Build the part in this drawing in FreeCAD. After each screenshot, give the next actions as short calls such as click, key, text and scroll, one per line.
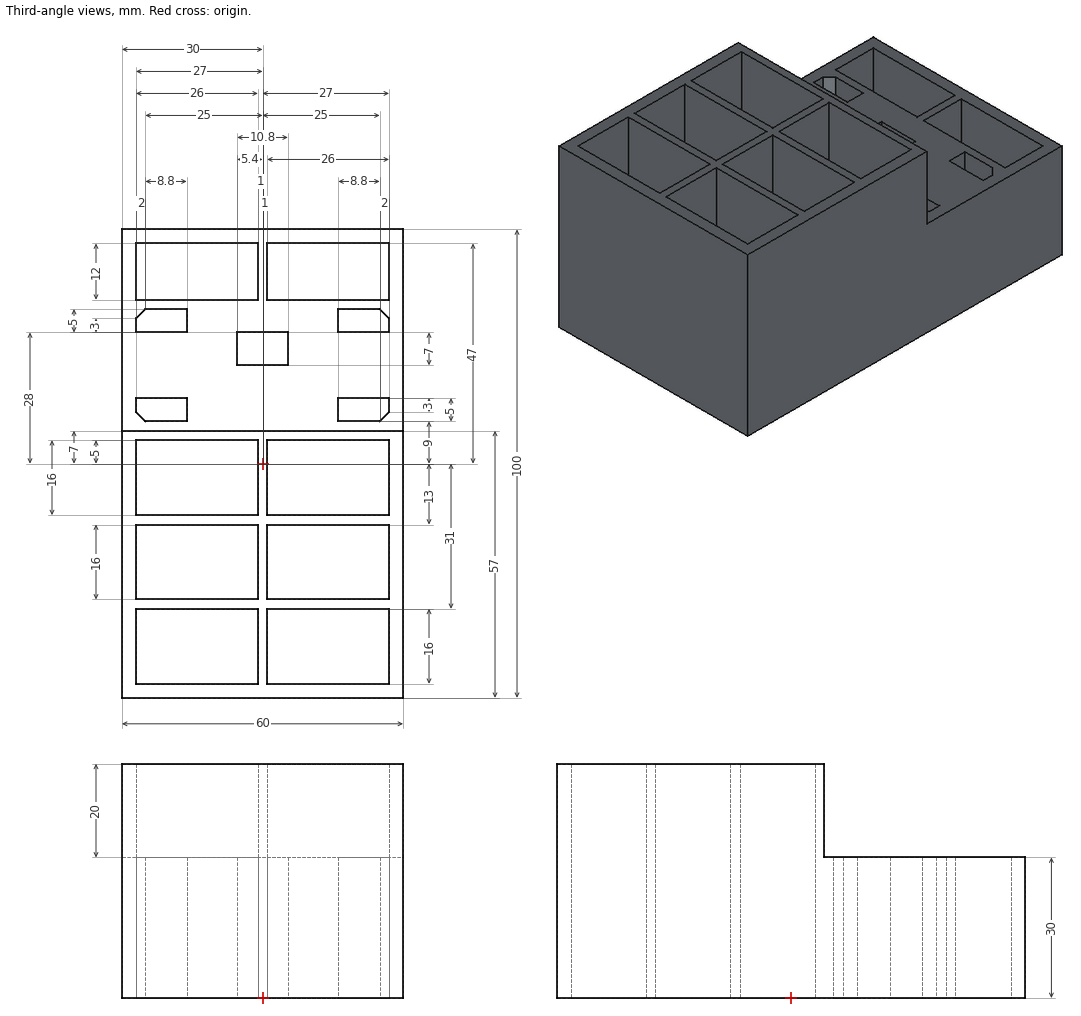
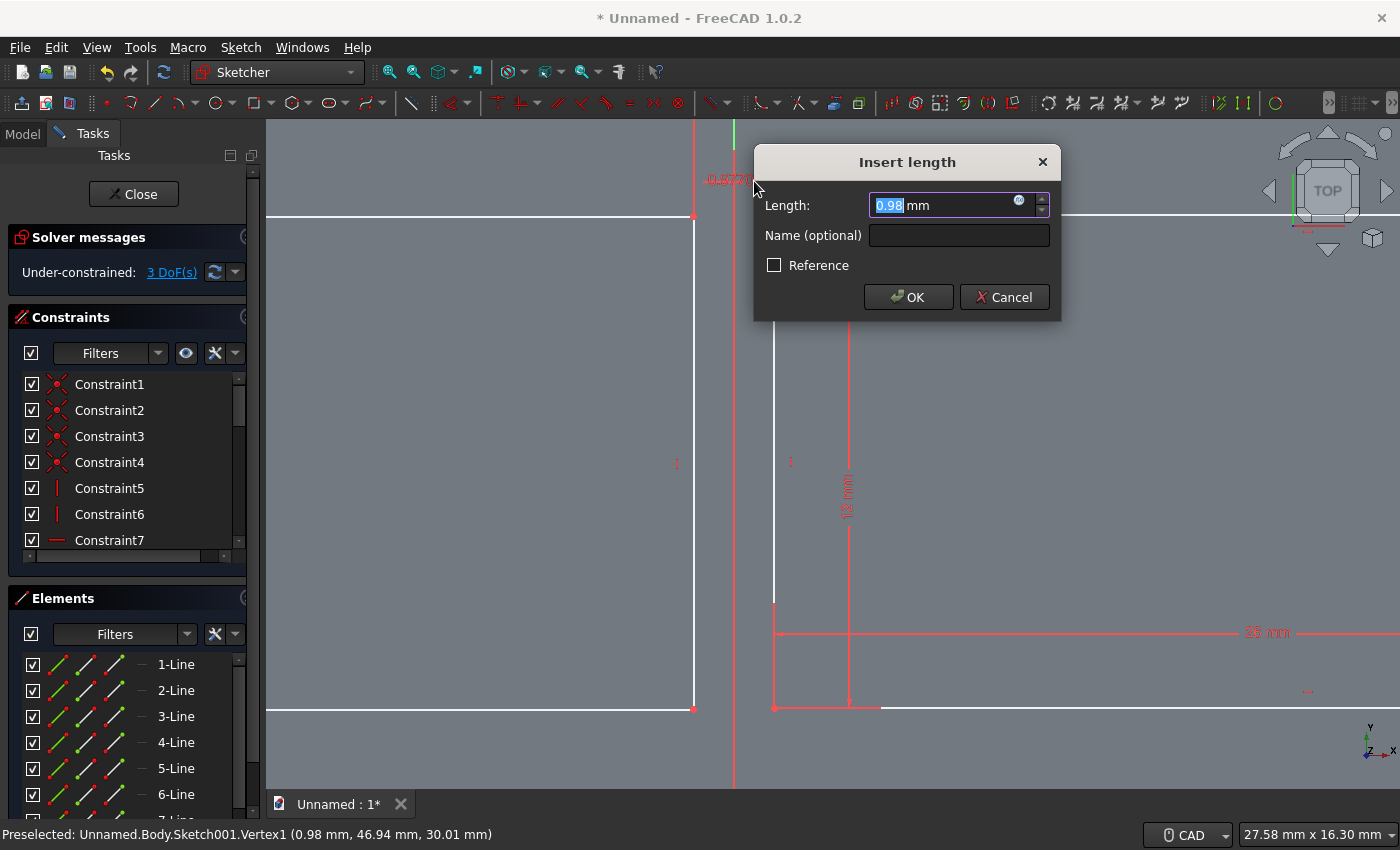
text(1)
key(Return)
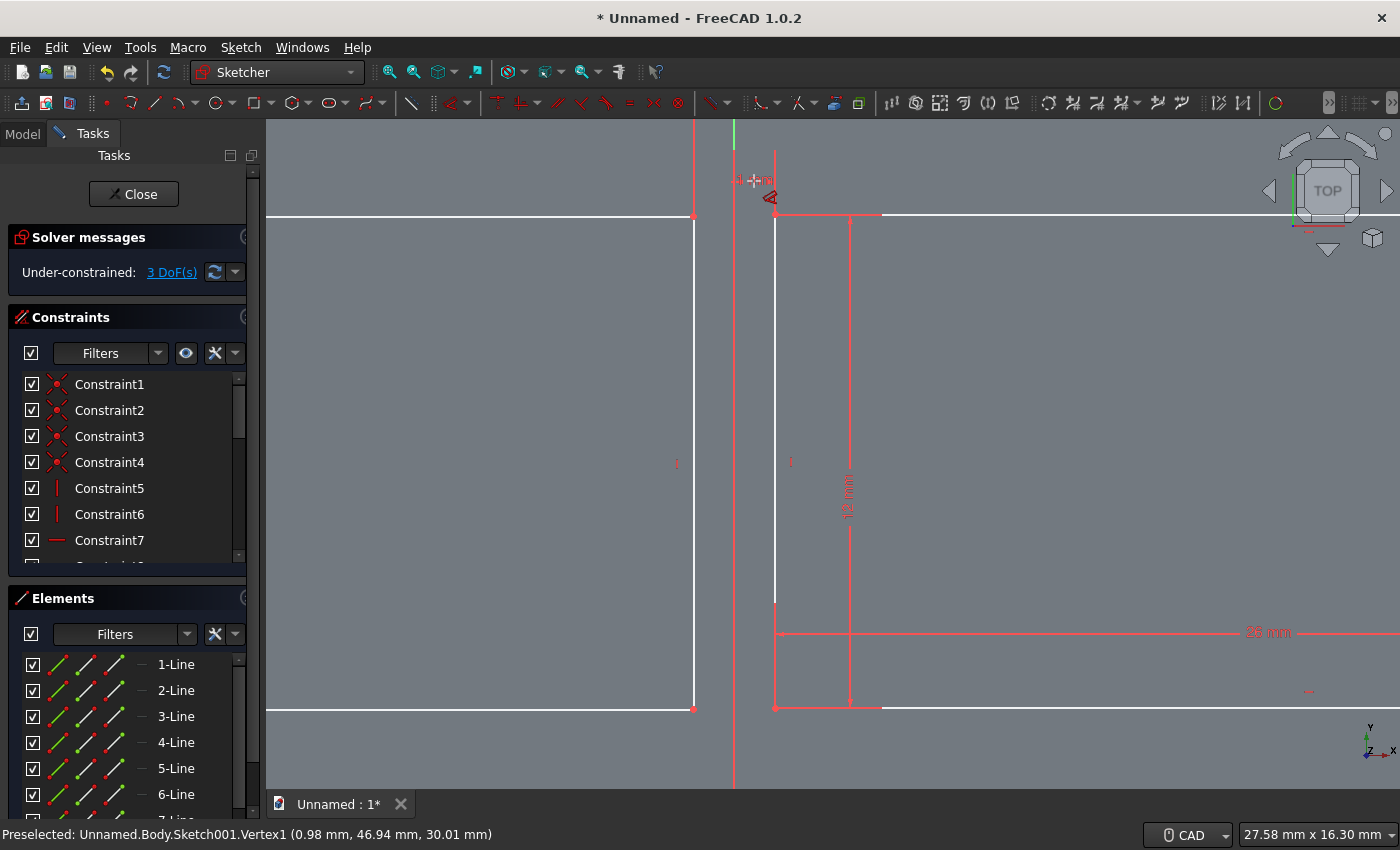
click(694, 710)
click(714, 676)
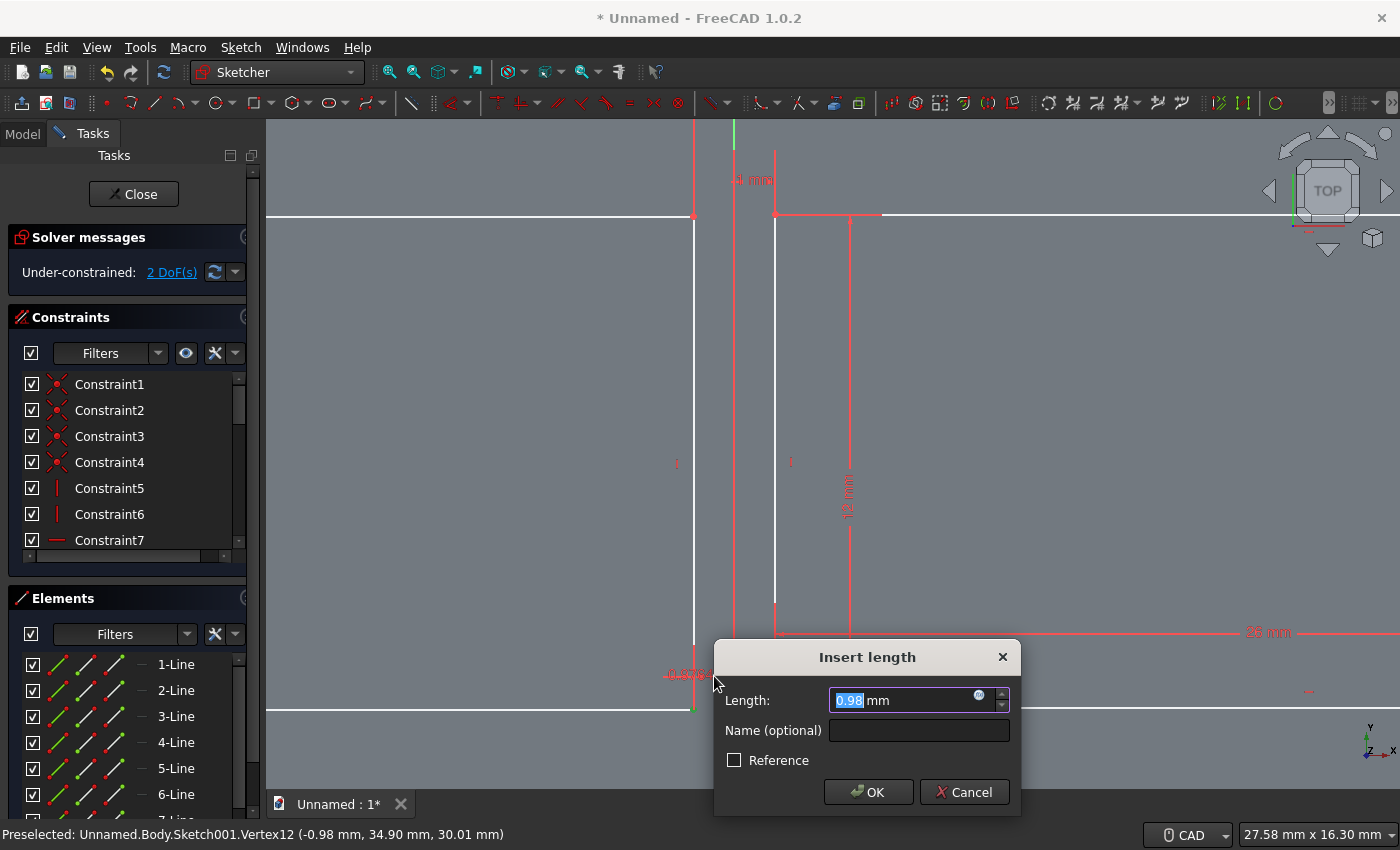
text(1)
key(Return)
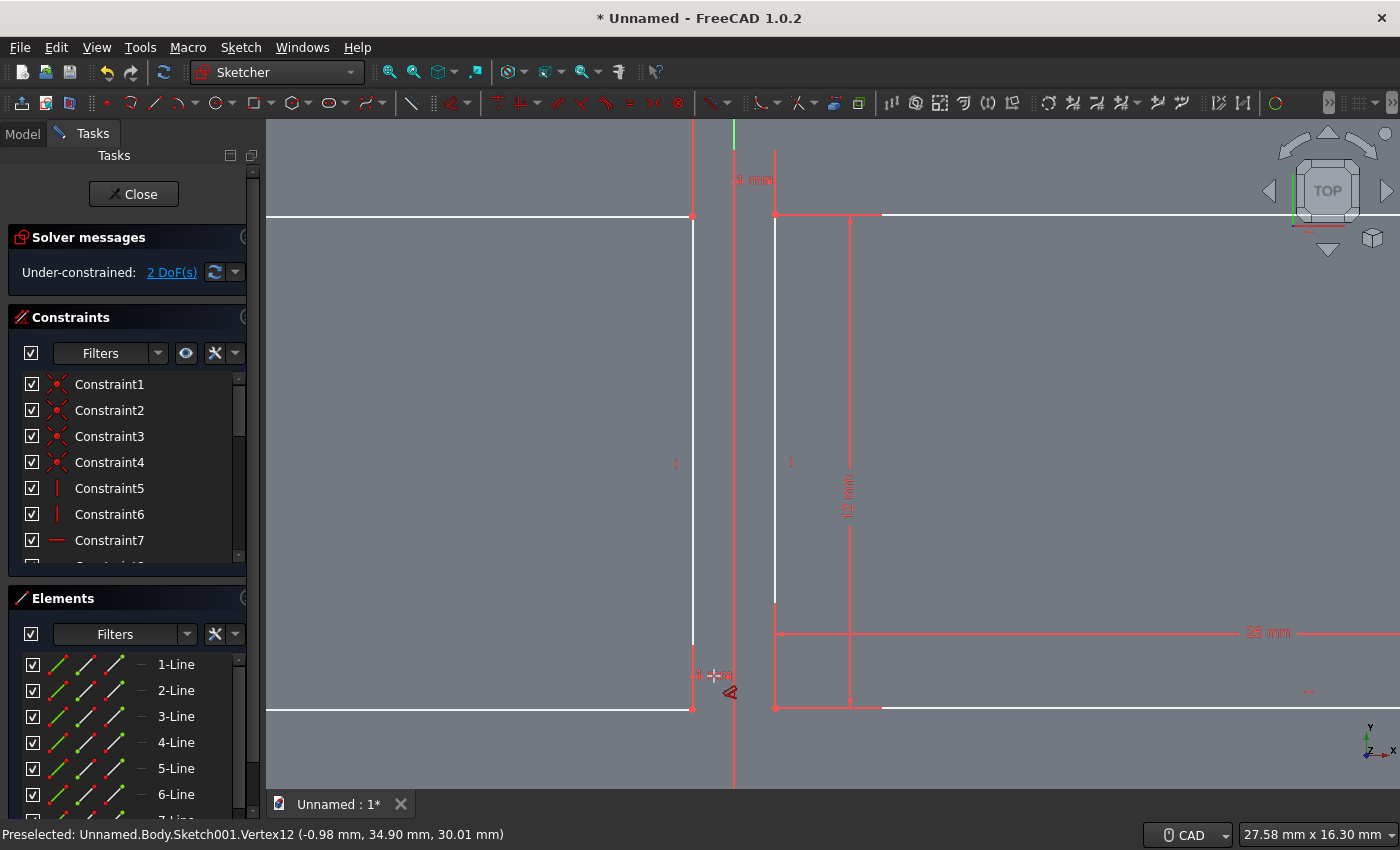
scroll(774, 217, down, 7)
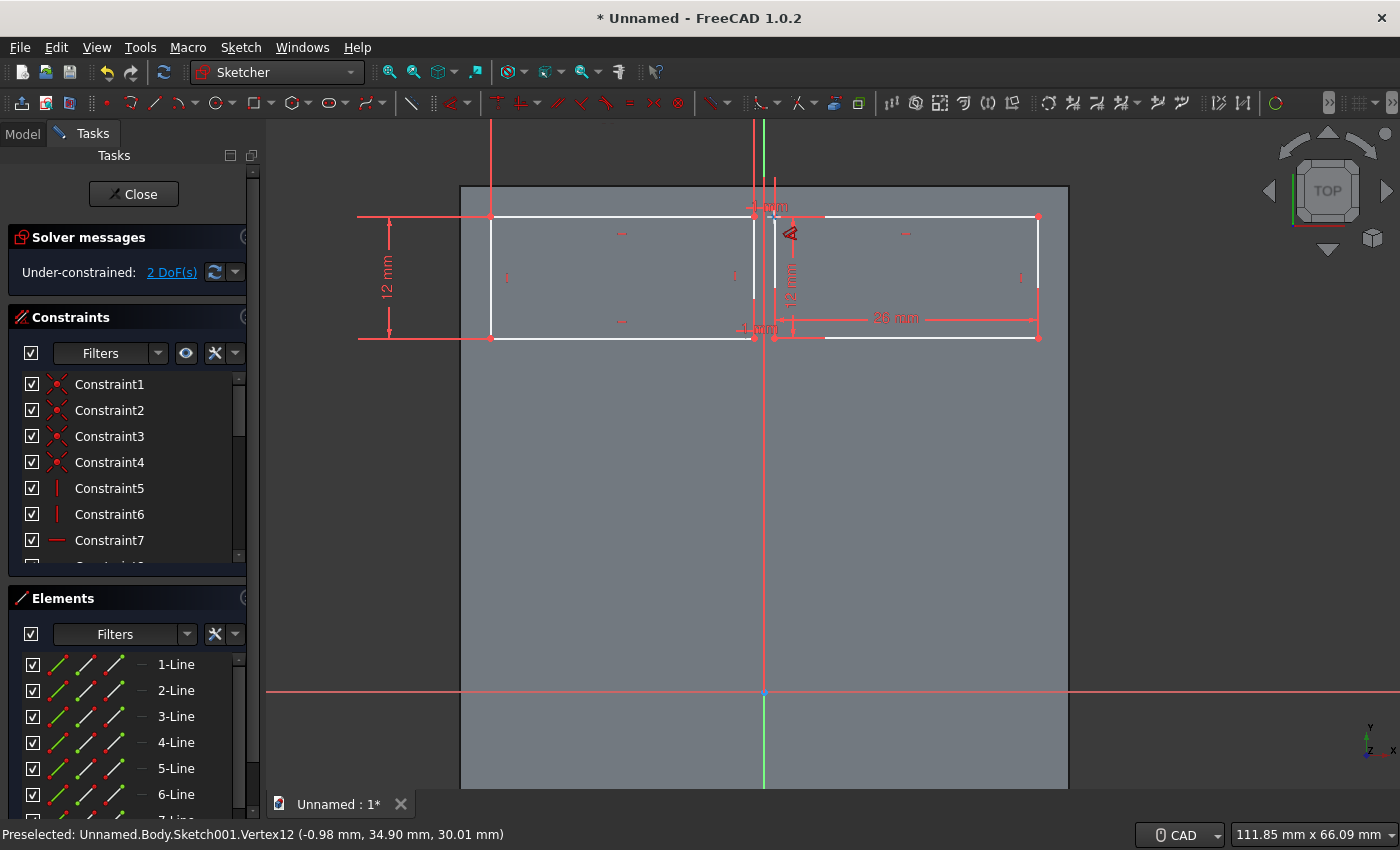
click(775, 217)
click(809, 455)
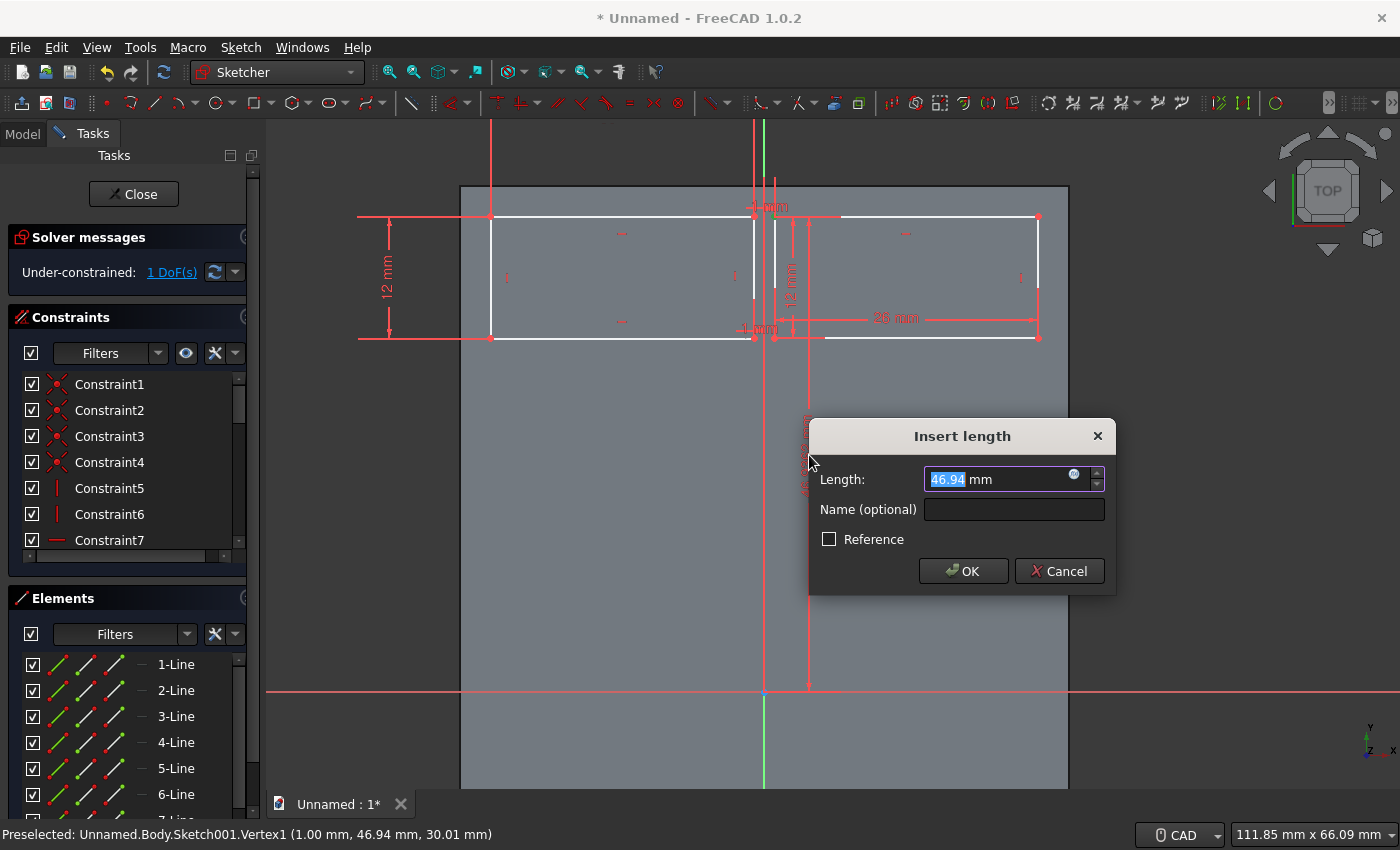
text(47)
key(Return)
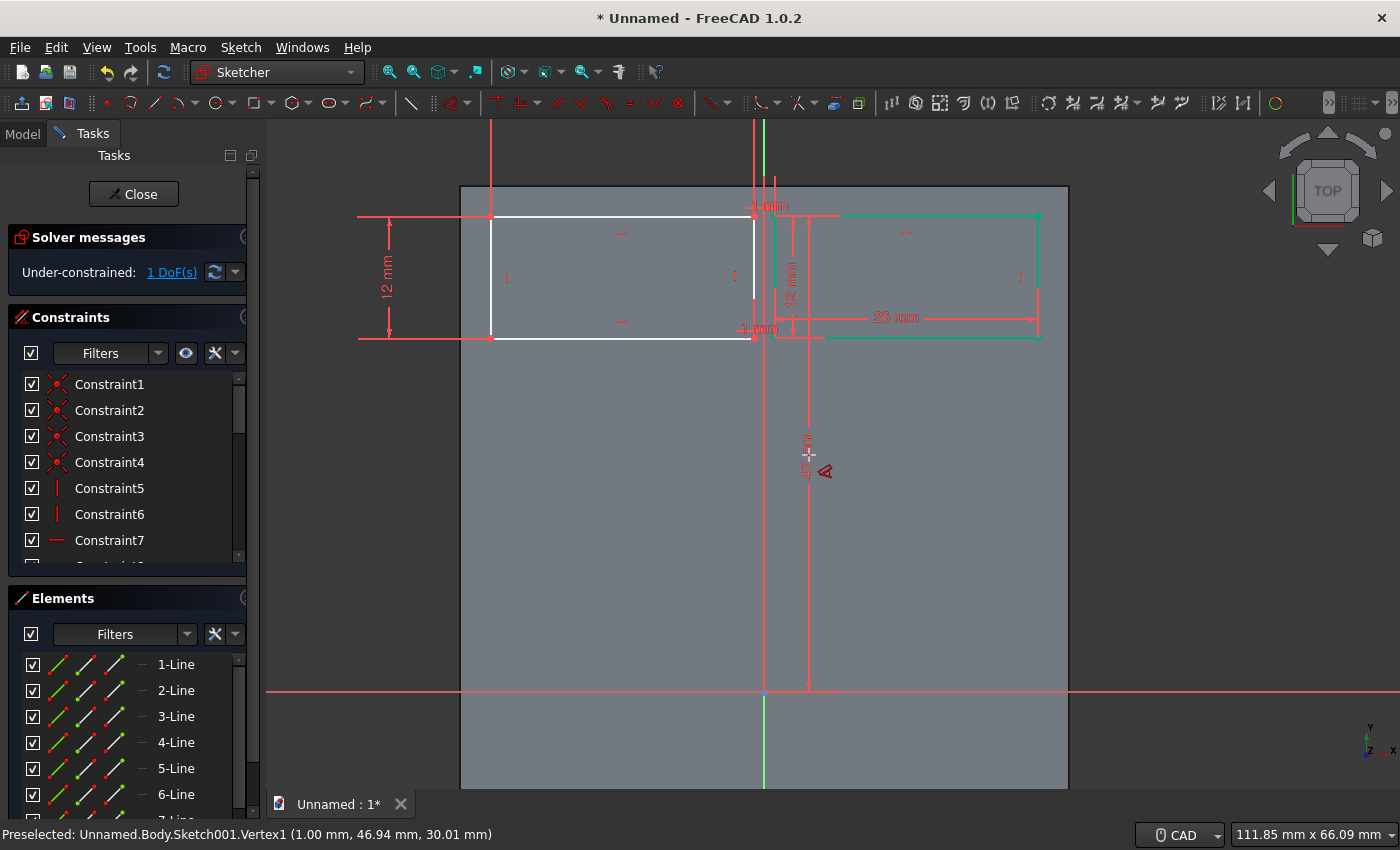
click(491, 217)
click(457, 455)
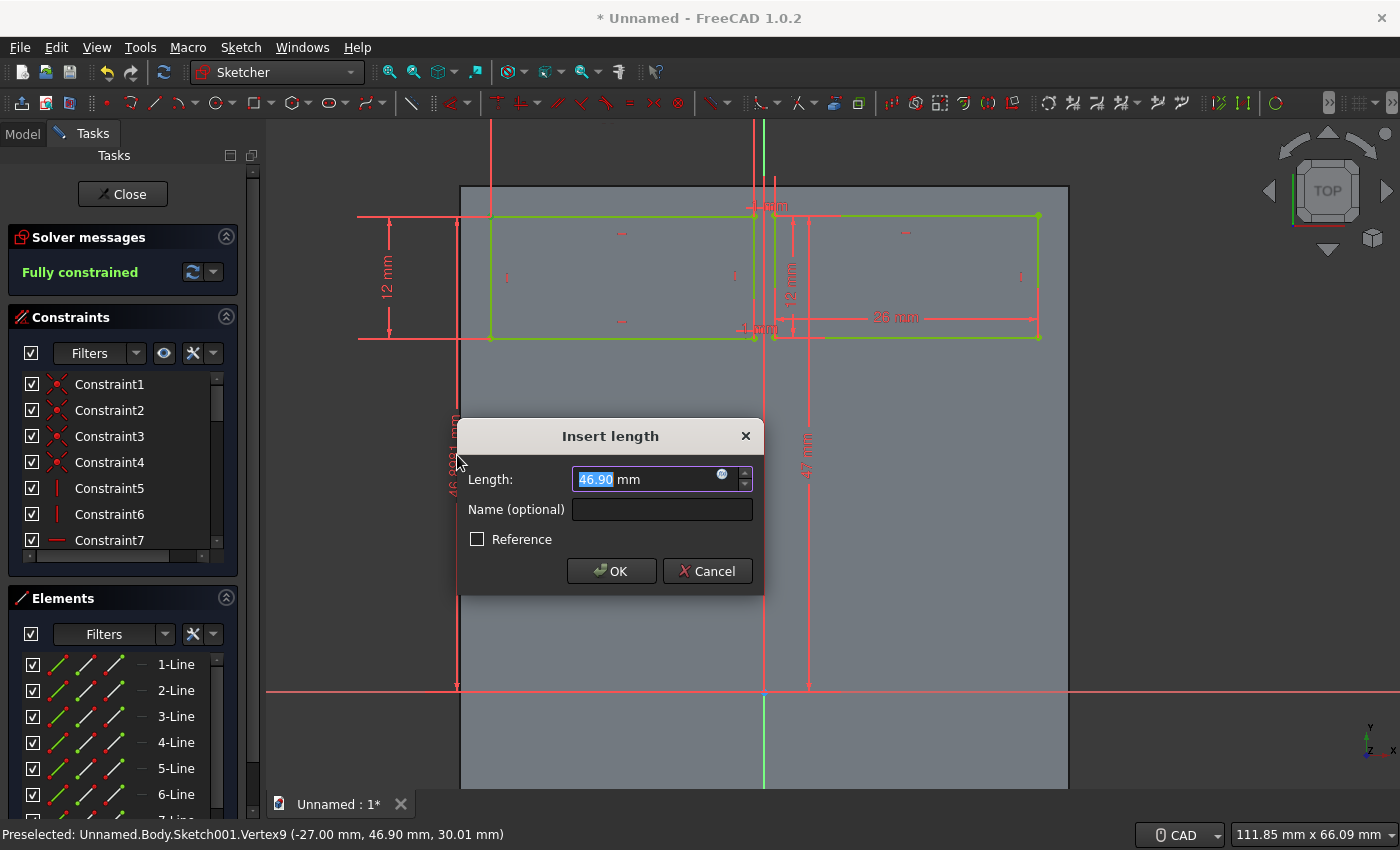
text(47)
key(Return)
key(Escape)